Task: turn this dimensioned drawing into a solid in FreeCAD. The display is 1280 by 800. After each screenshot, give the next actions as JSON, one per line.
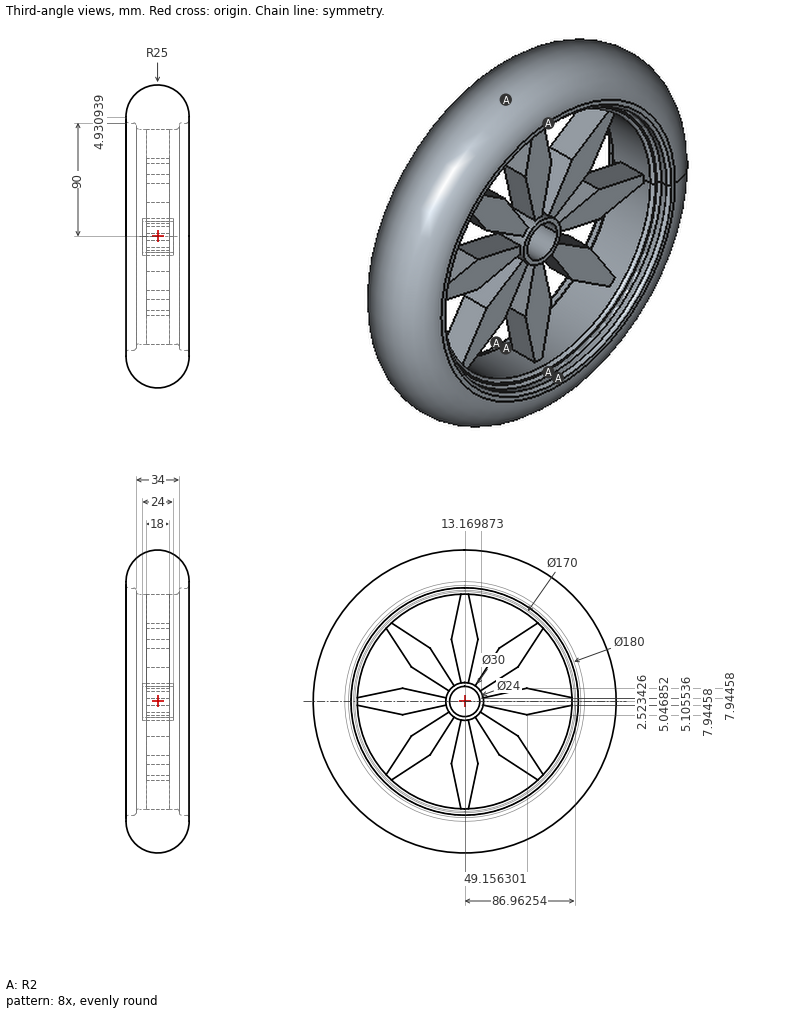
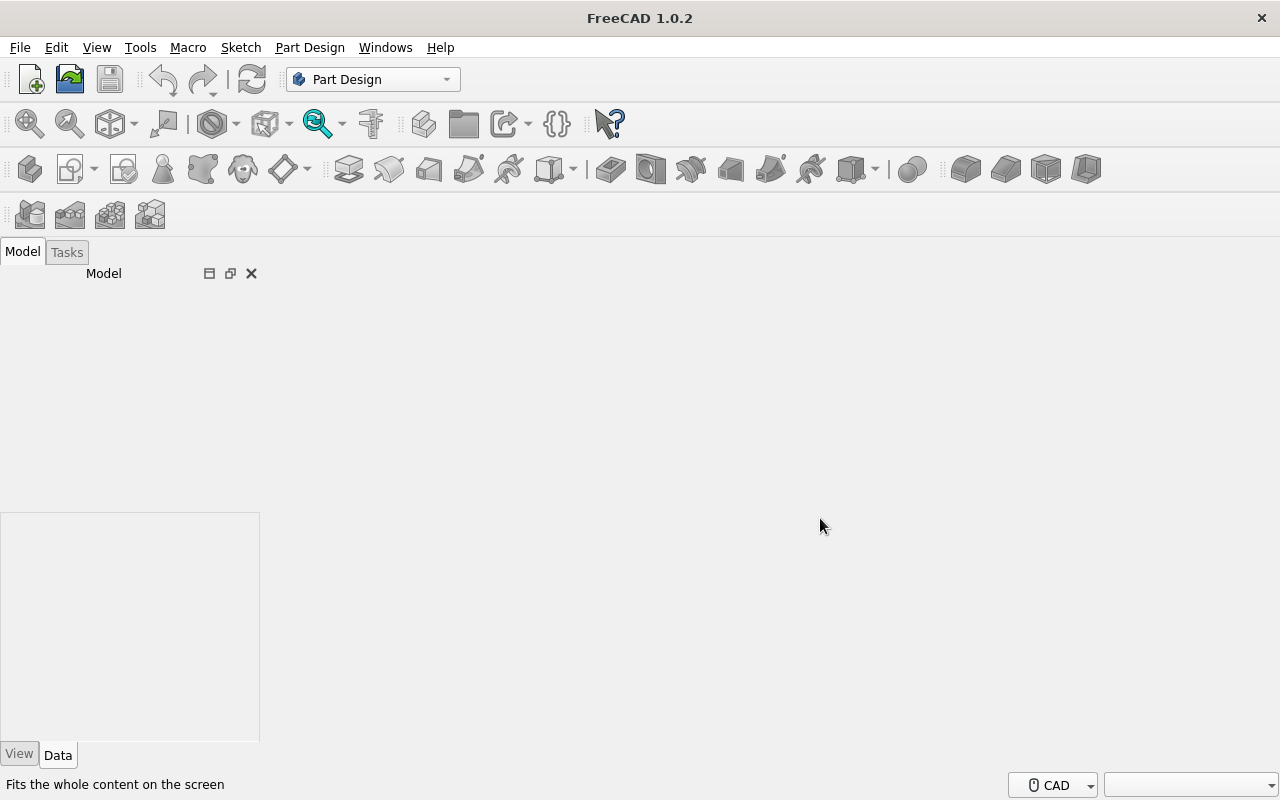
{"action": "left_click", "coordinate": [30, 80]}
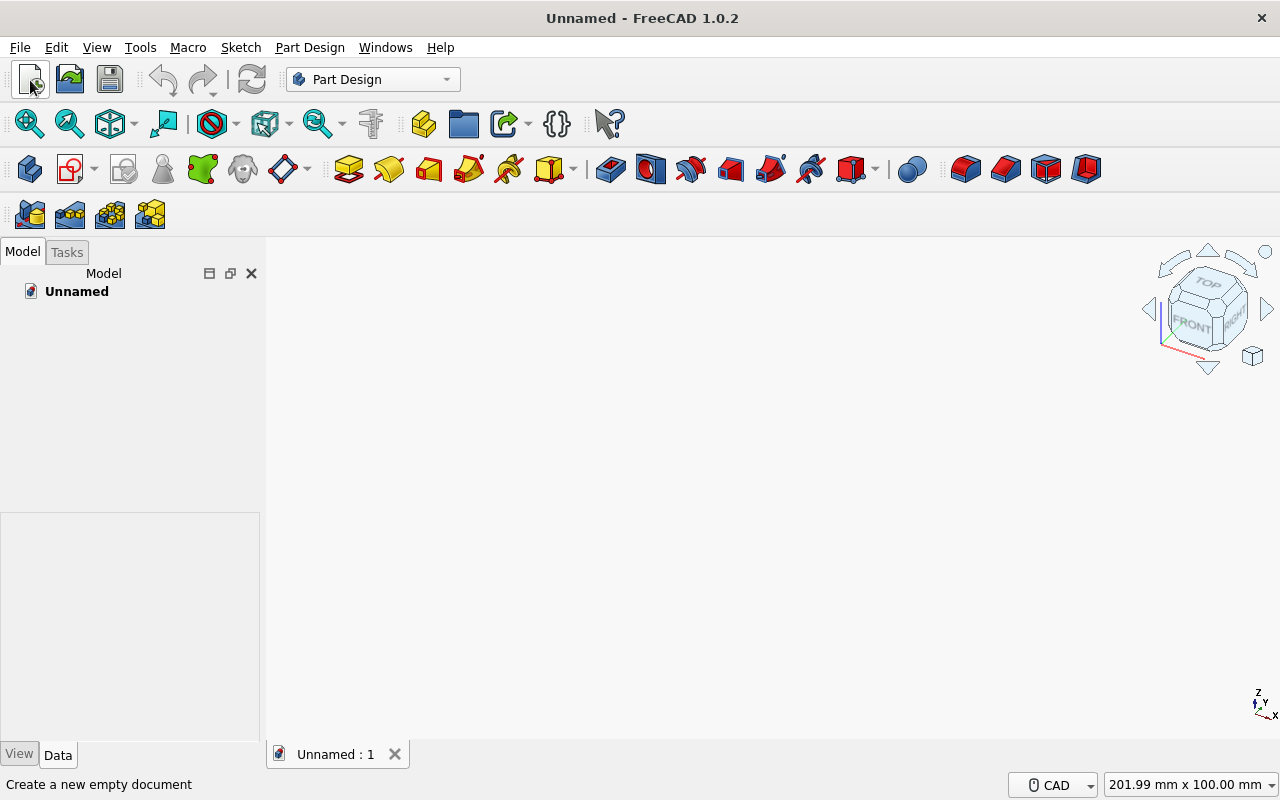
{"action": "left_click", "coordinate": [70, 170]}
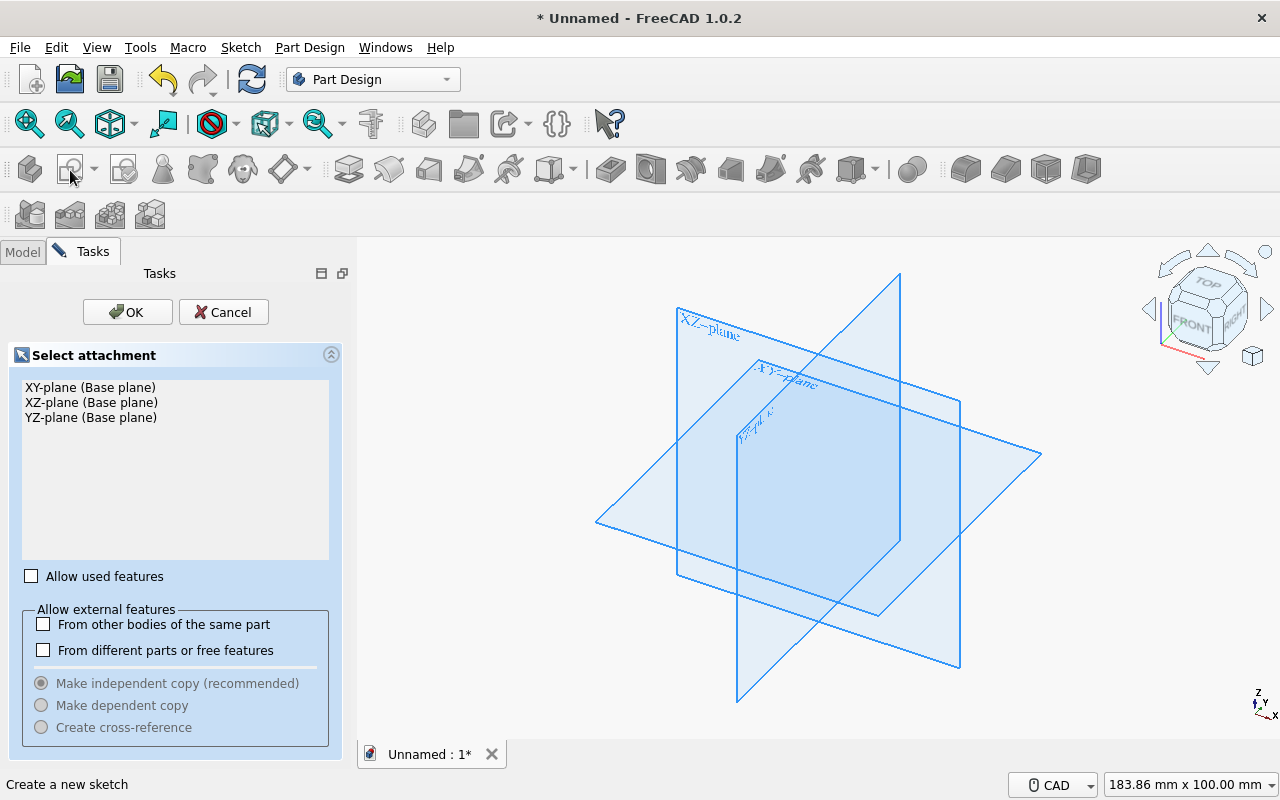
{"action": "left_click", "coordinate": [82, 388]}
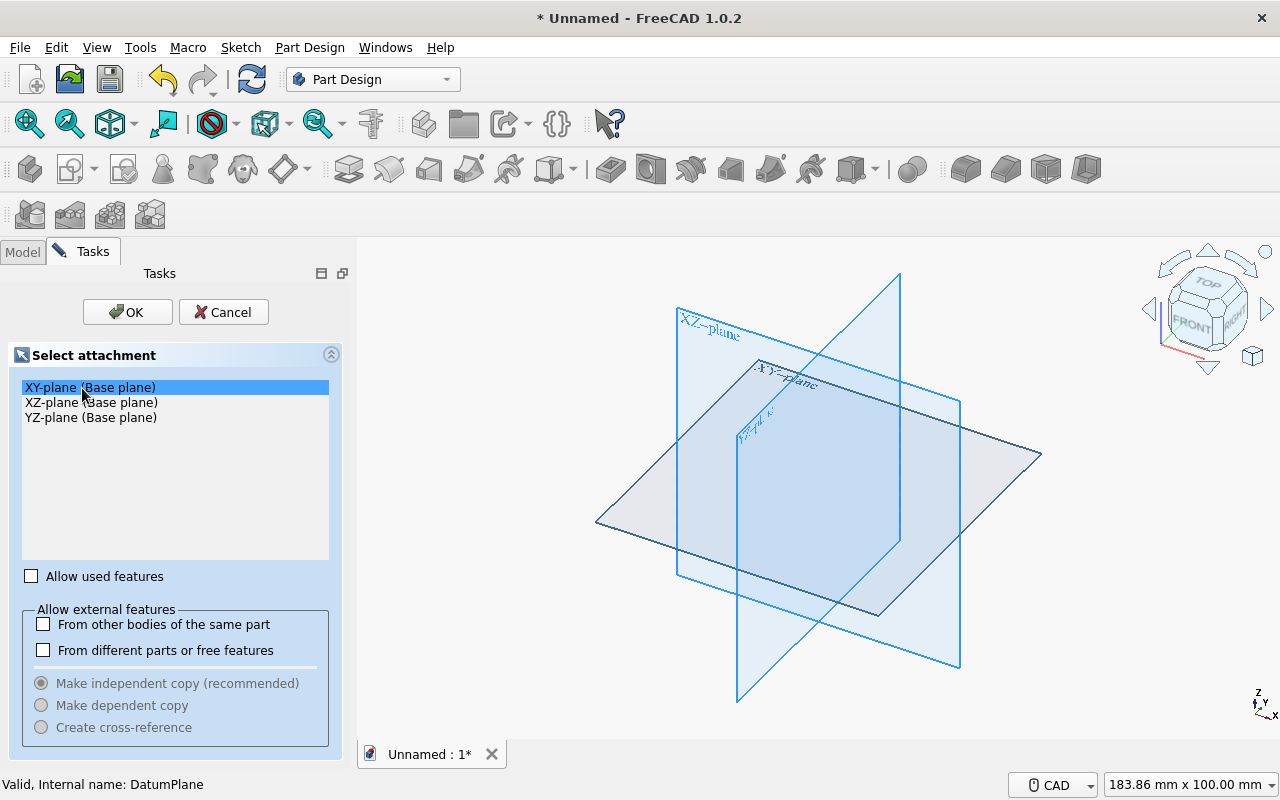
{"action": "left_click", "coordinate": [128, 312]}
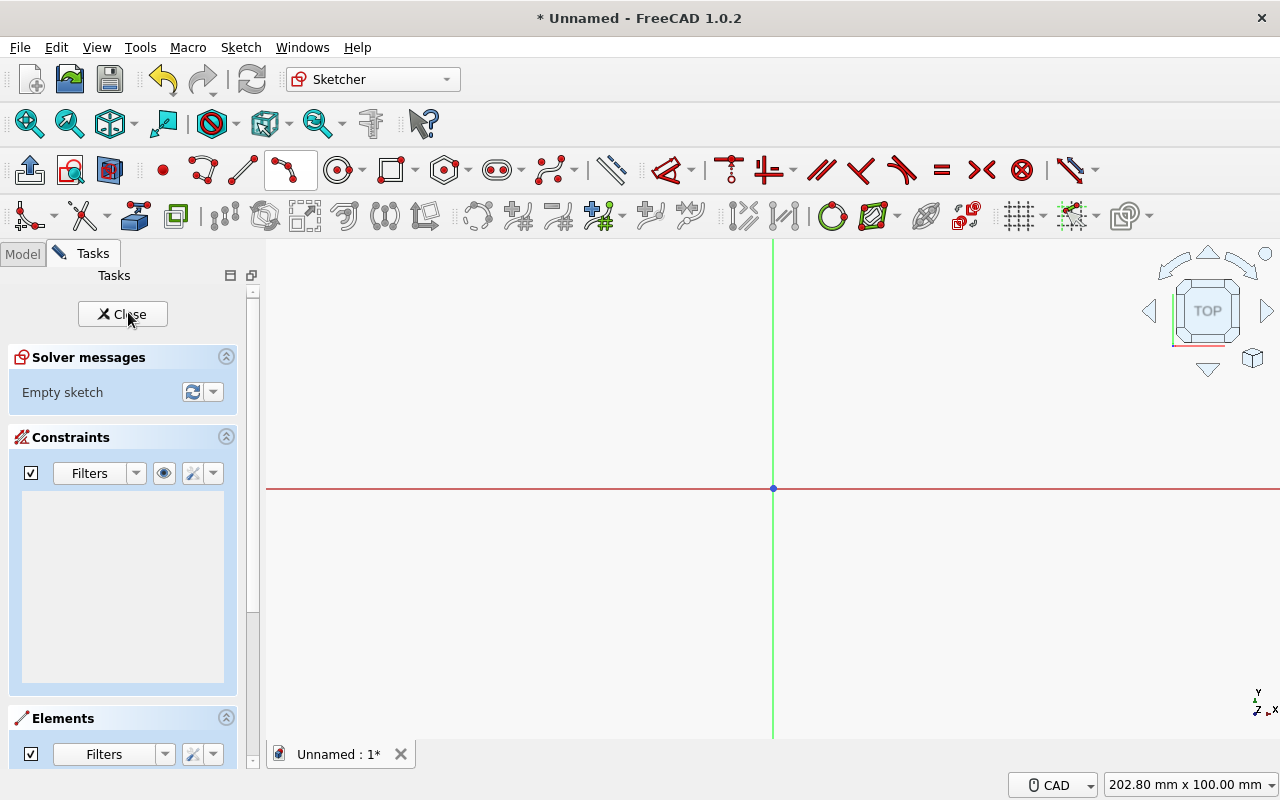
{"action": "scroll", "coordinate": [649, 711], "scroll_direction": "down", "scroll_amount": 4}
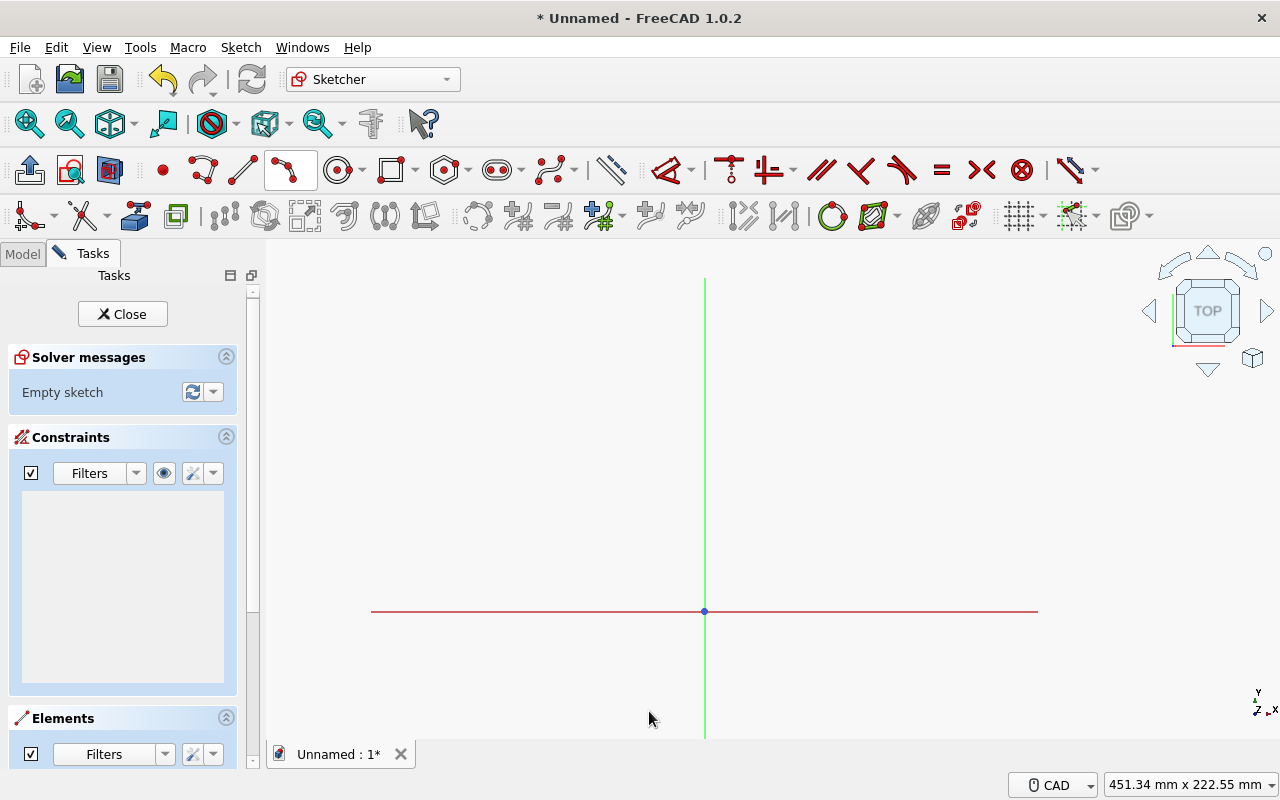
{"action": "key", "text": "g m"}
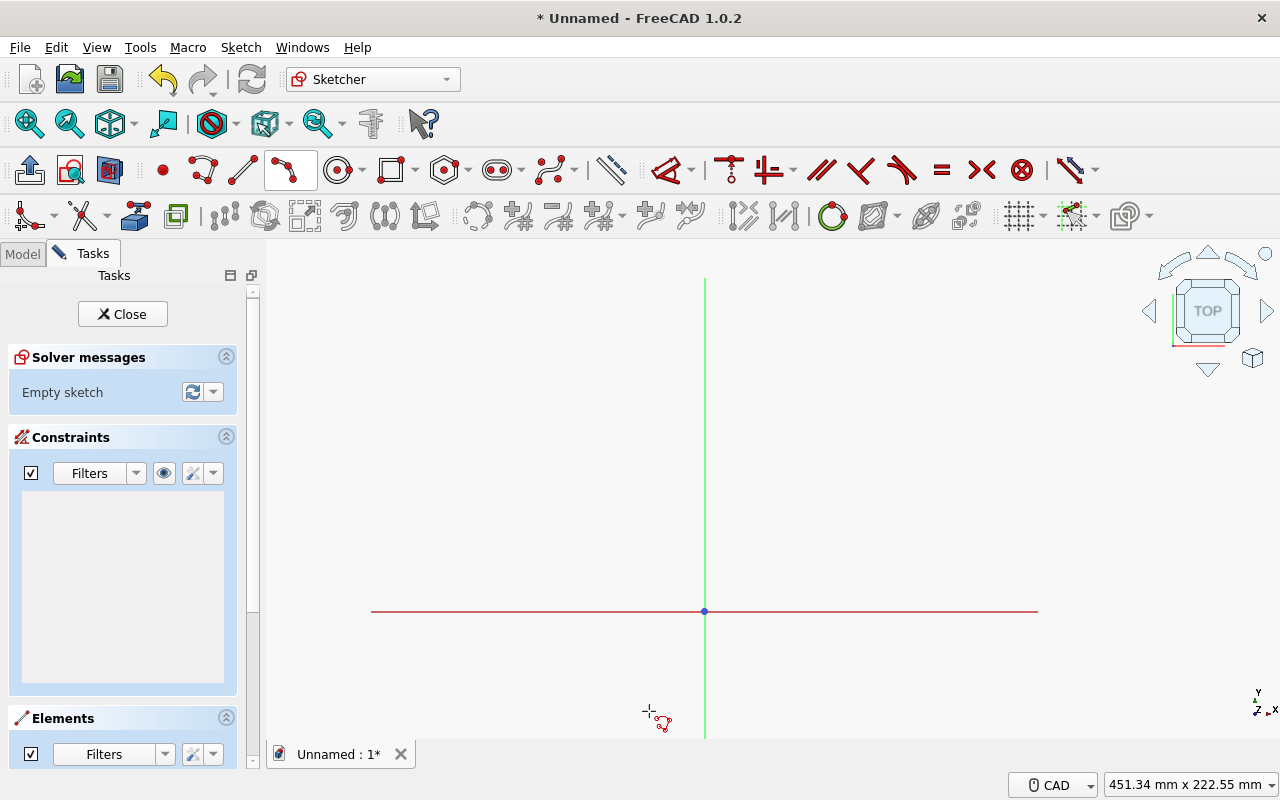
{"action": "left_click", "coordinate": [649, 398]}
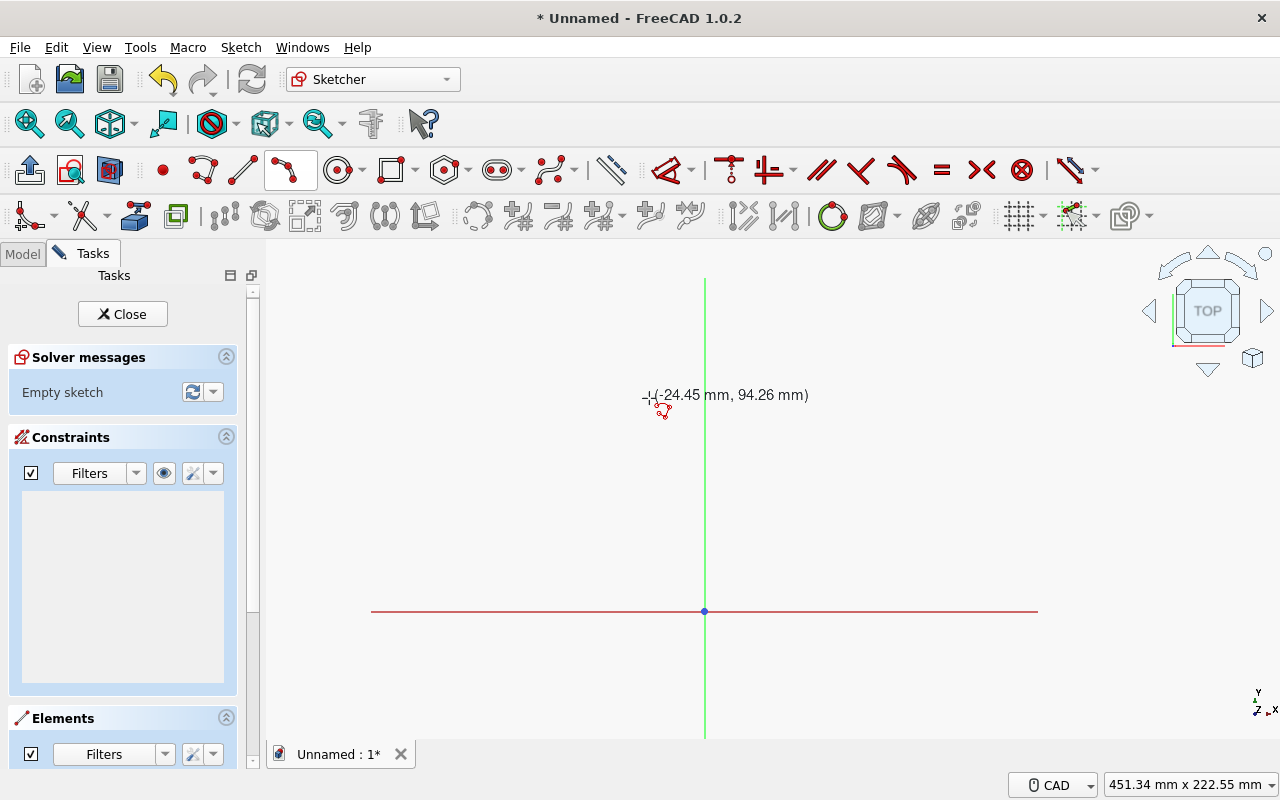
{"action": "scroll", "coordinate": [649, 410], "scroll_direction": "up", "scroll_amount": 2}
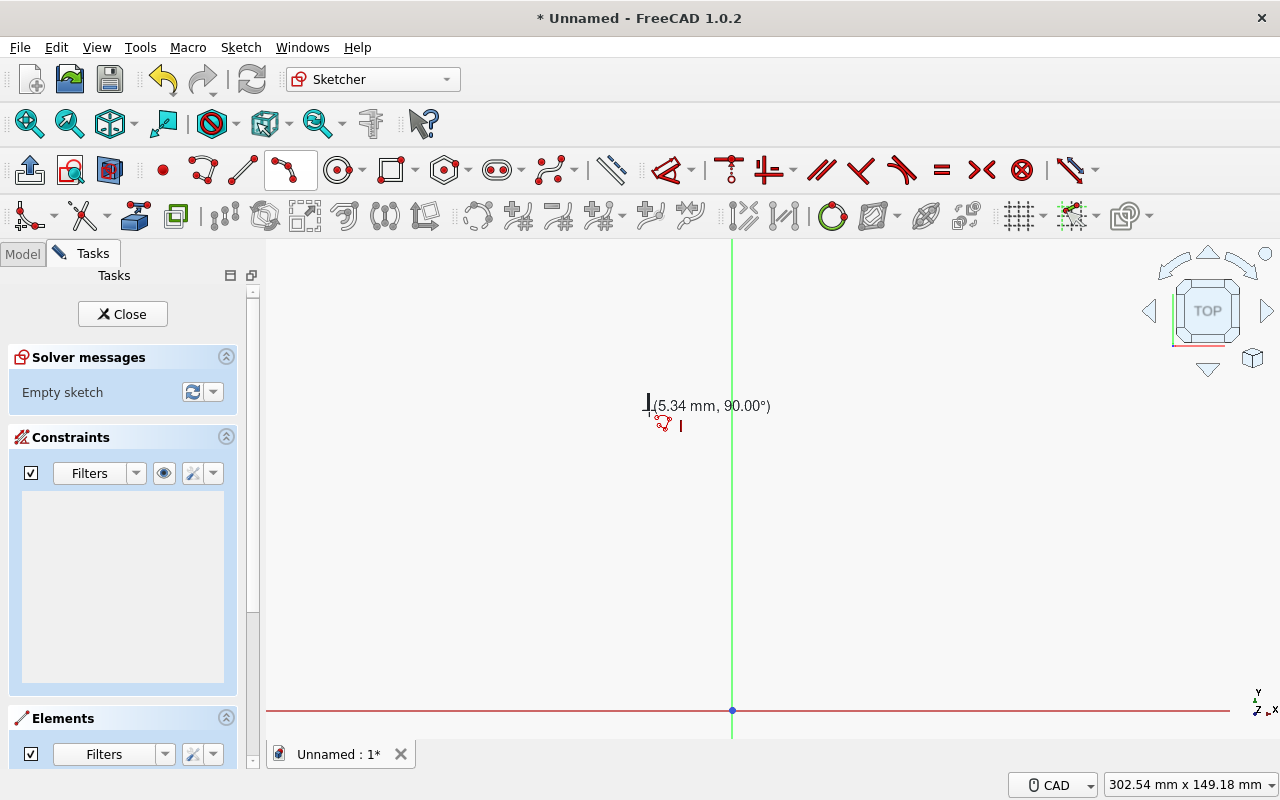
{"action": "left_click", "coordinate": [649, 409]}
{"action": "left_click", "coordinate": [816, 409]}
{"action": "left_click", "coordinate": [816, 393]}
{"action": "right_click", "coordinate": [816, 393]}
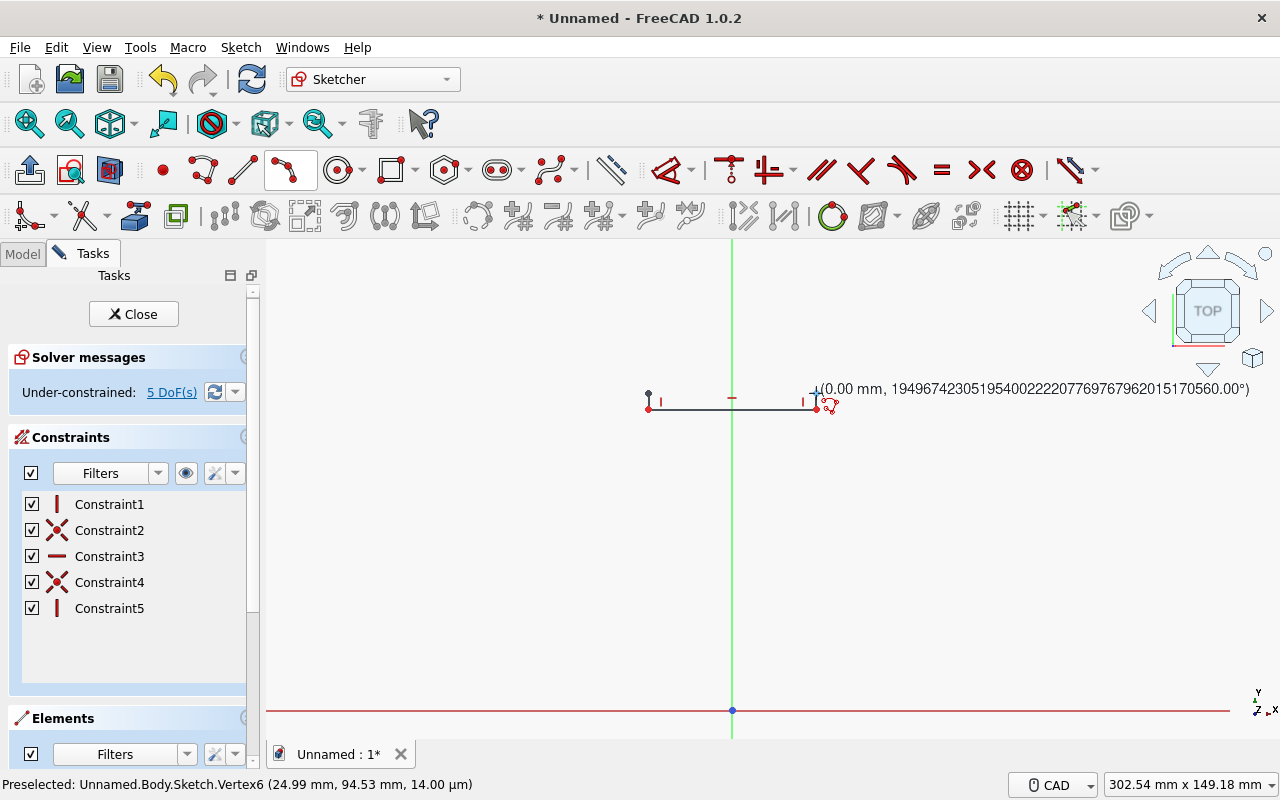
{"action": "left_click", "coordinate": [284, 170]}